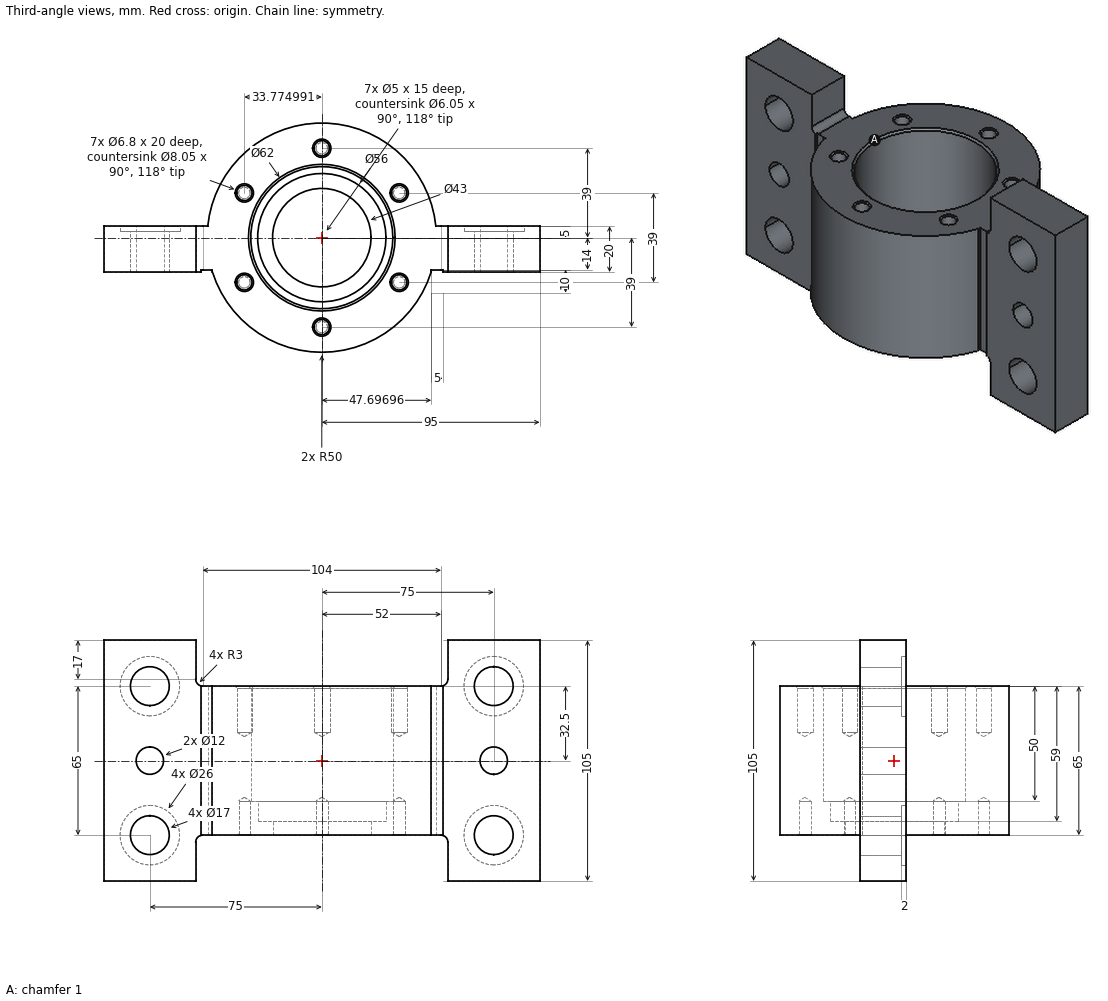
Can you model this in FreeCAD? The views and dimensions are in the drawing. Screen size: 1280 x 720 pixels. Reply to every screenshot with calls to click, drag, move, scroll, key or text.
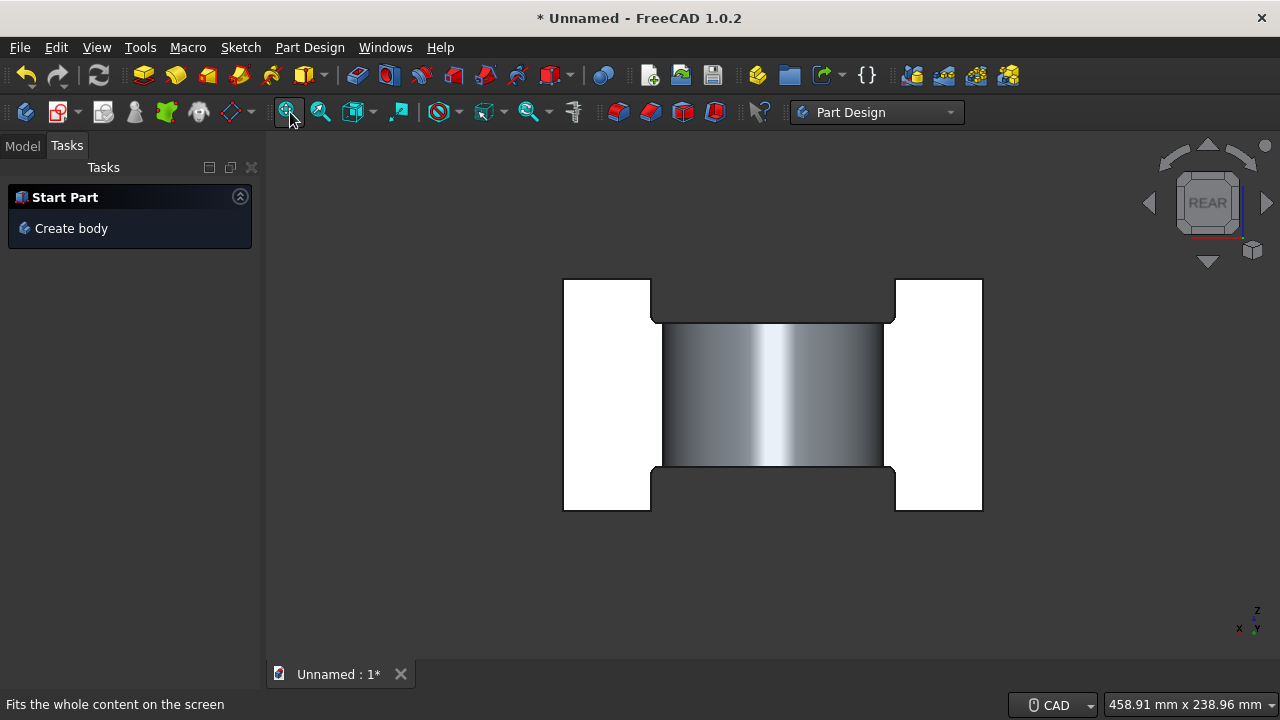
click(933, 361)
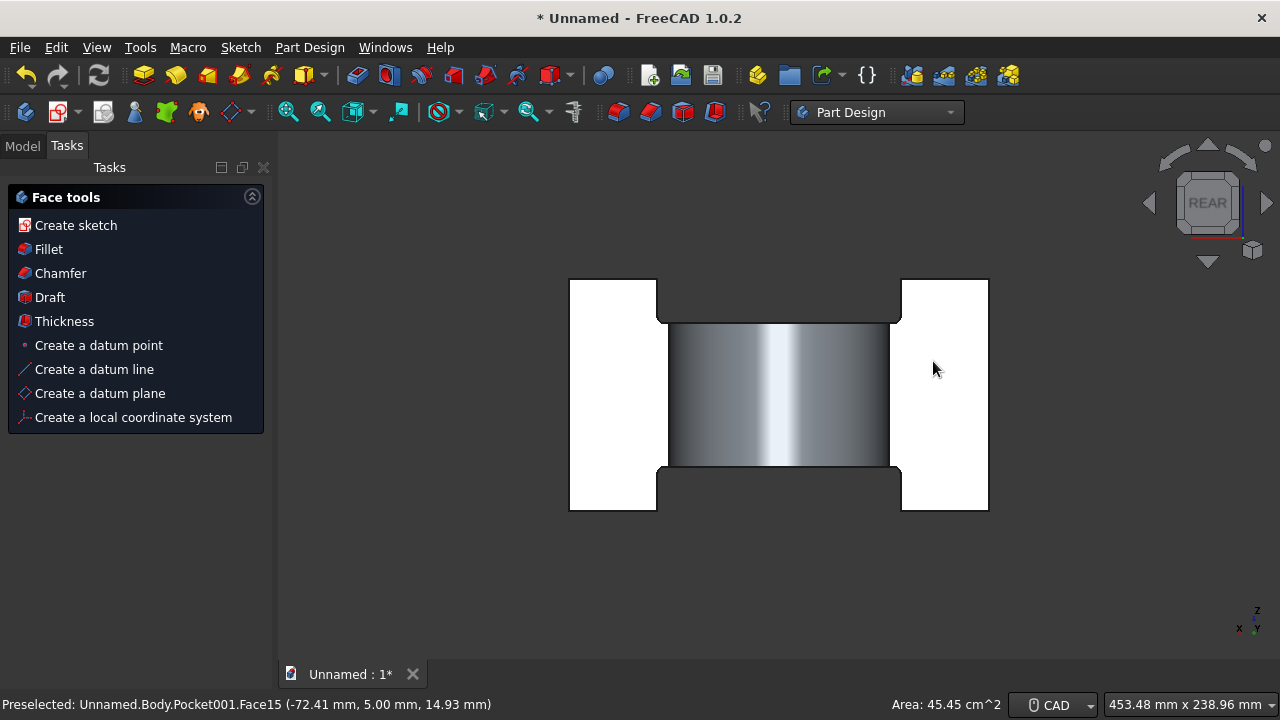
click(58, 112)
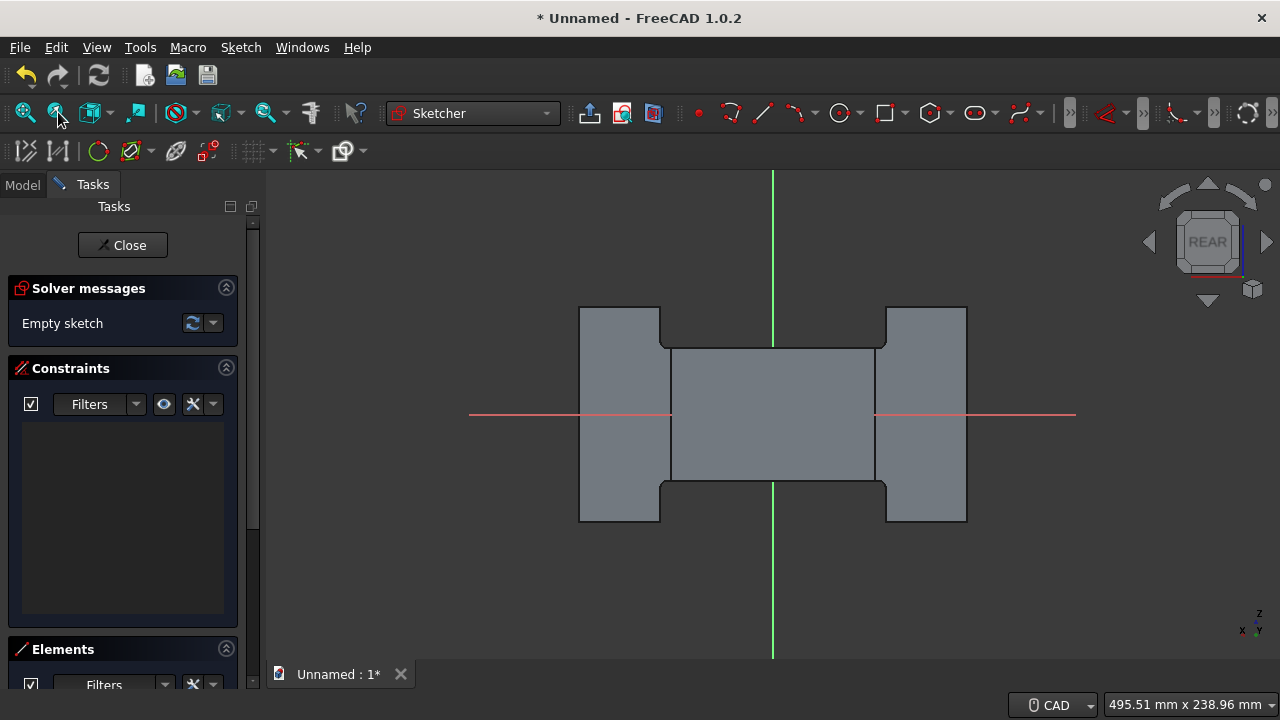
click(654, 114)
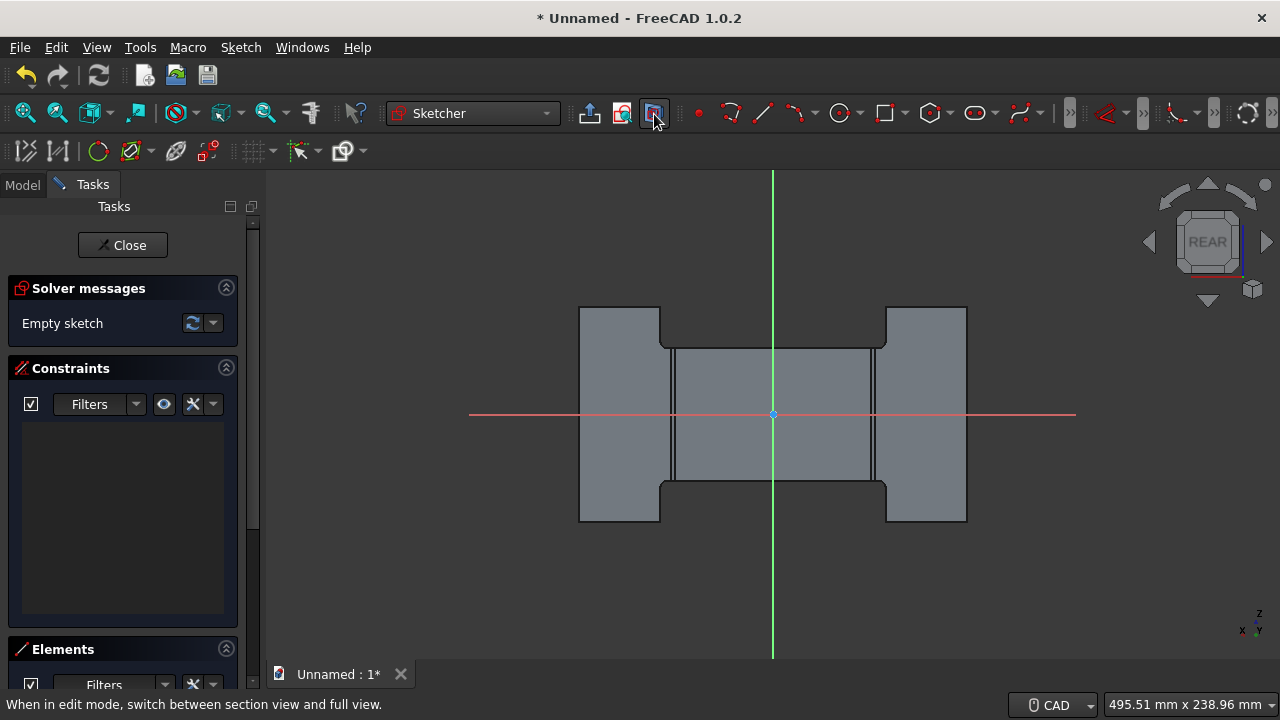
scroll(856, 415, up, 3)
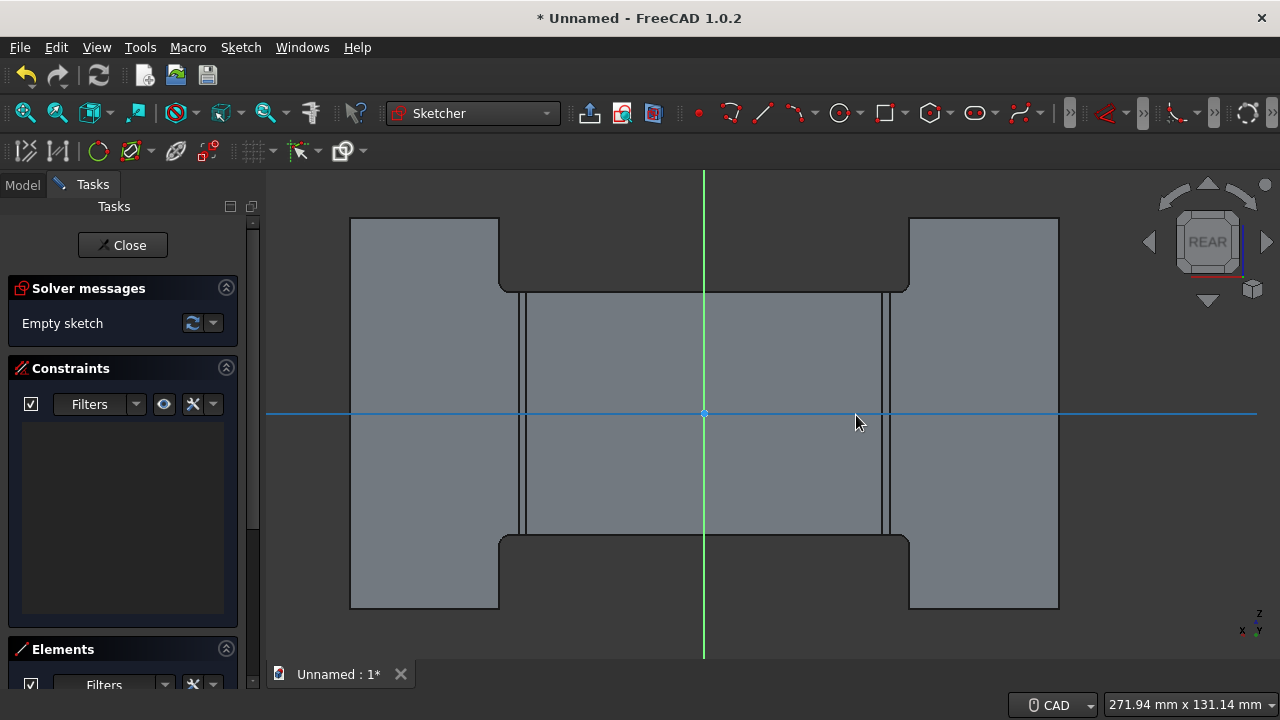
click(840, 114)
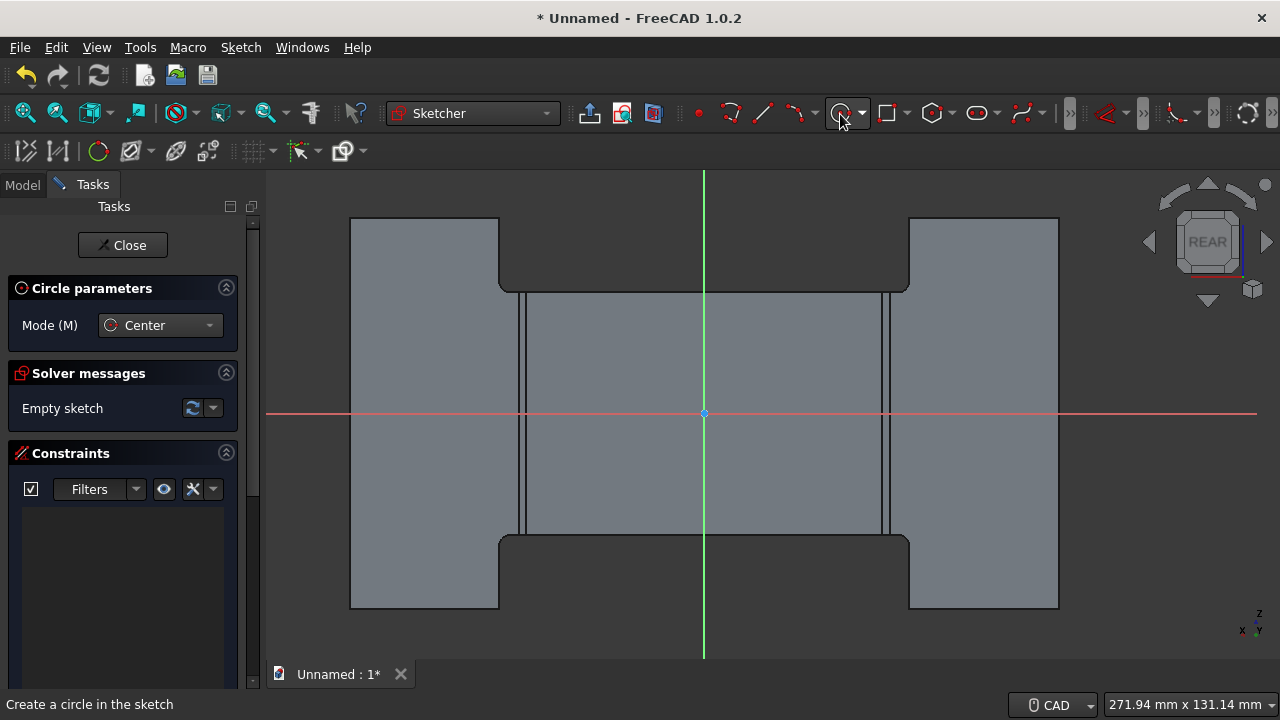
click(984, 535)
click(1006, 512)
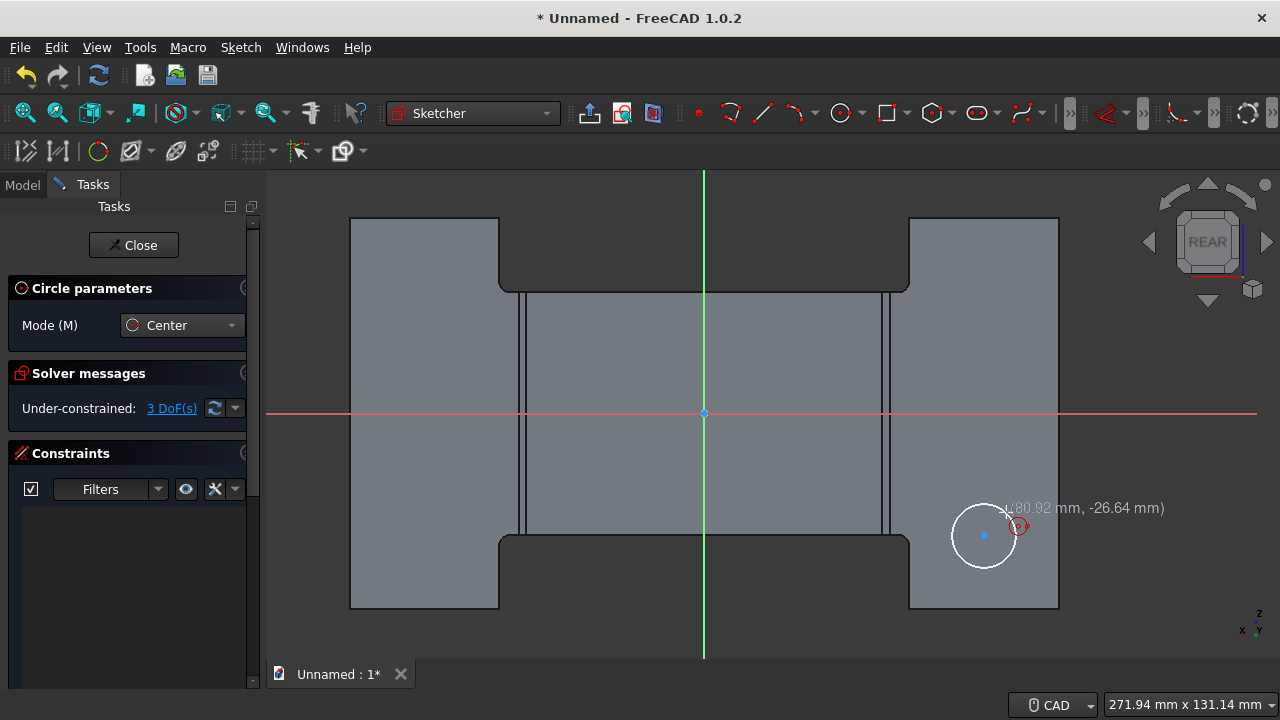
click(984, 292)
click(1006, 270)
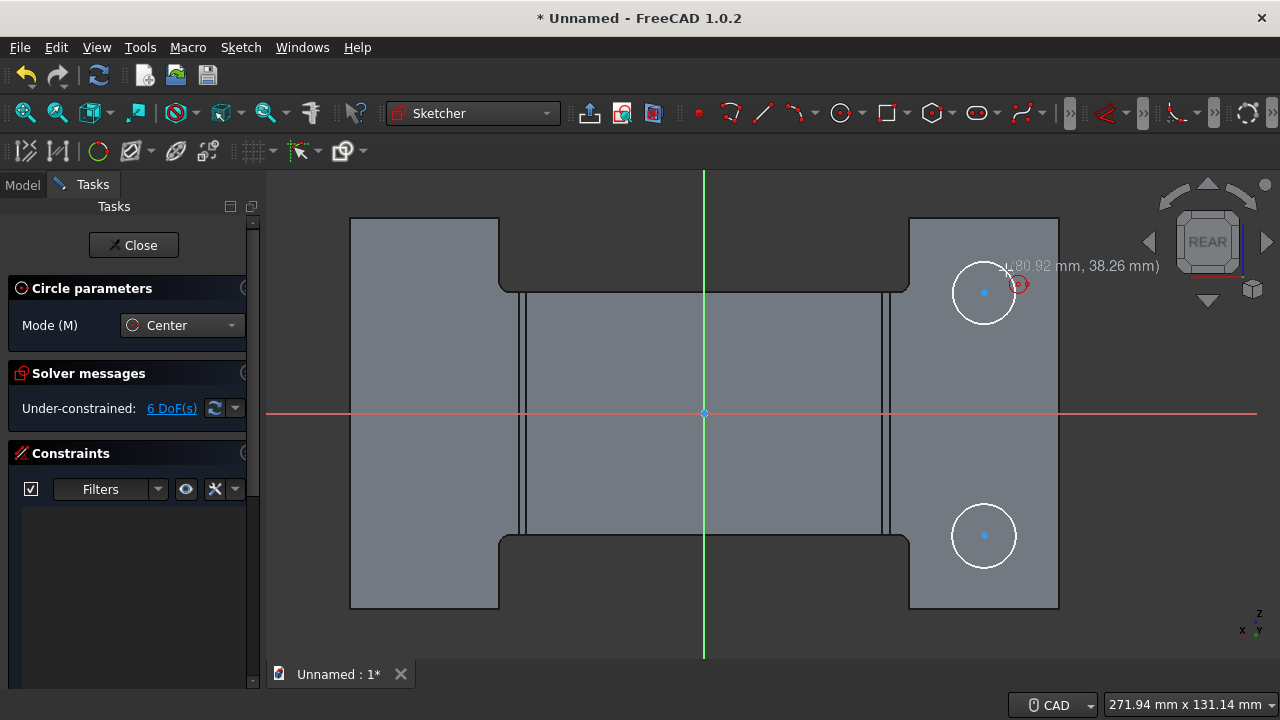
click(425, 292)
click(447, 270)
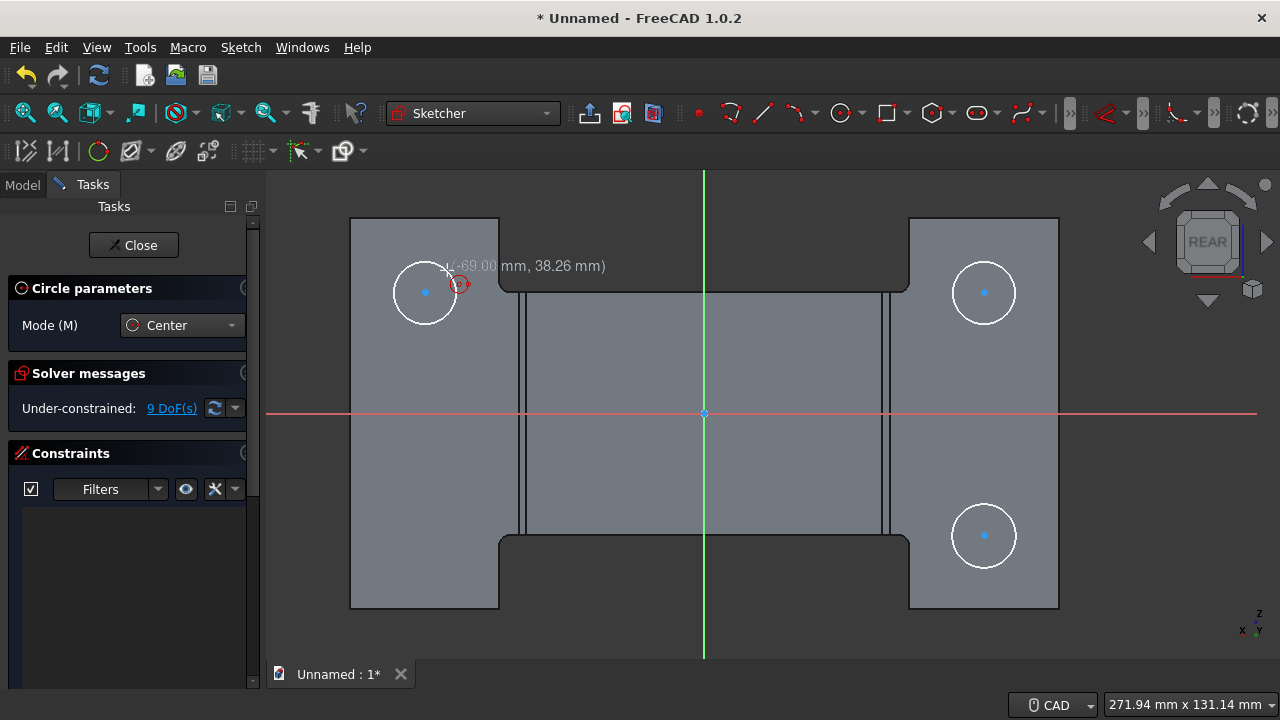
click(425, 535)
click(447, 512)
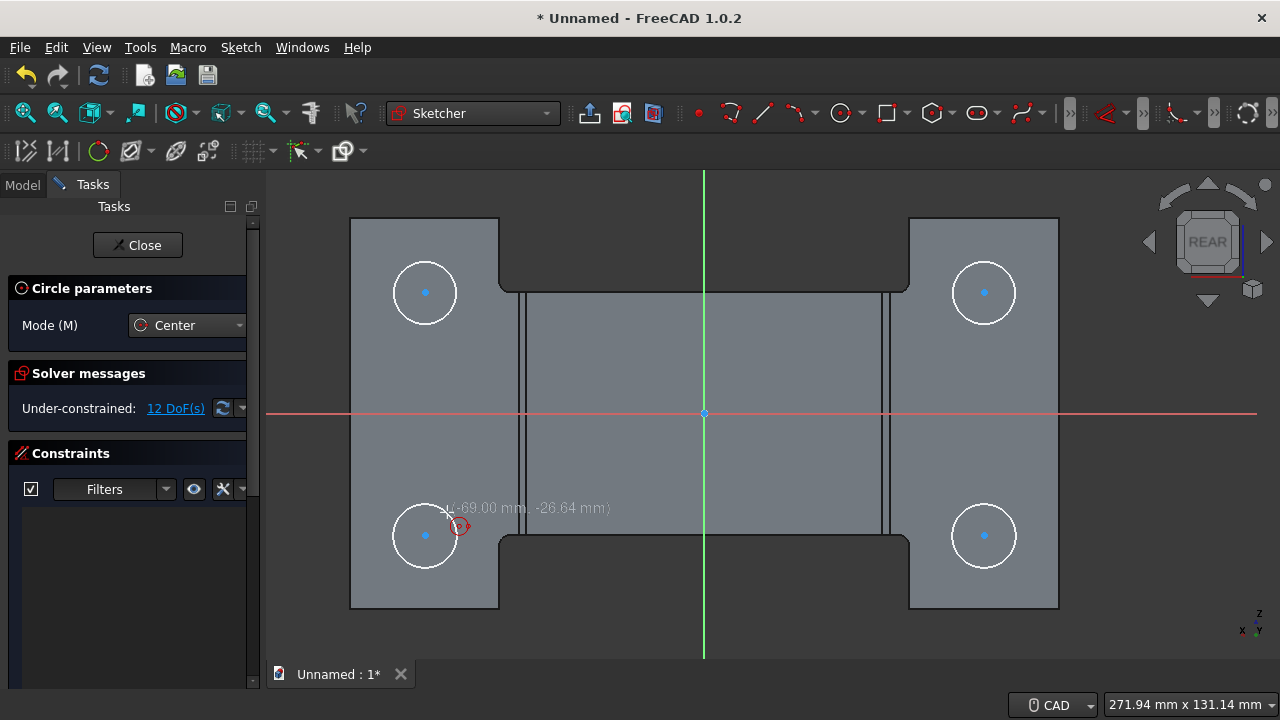
click(984, 414)
click(1000, 398)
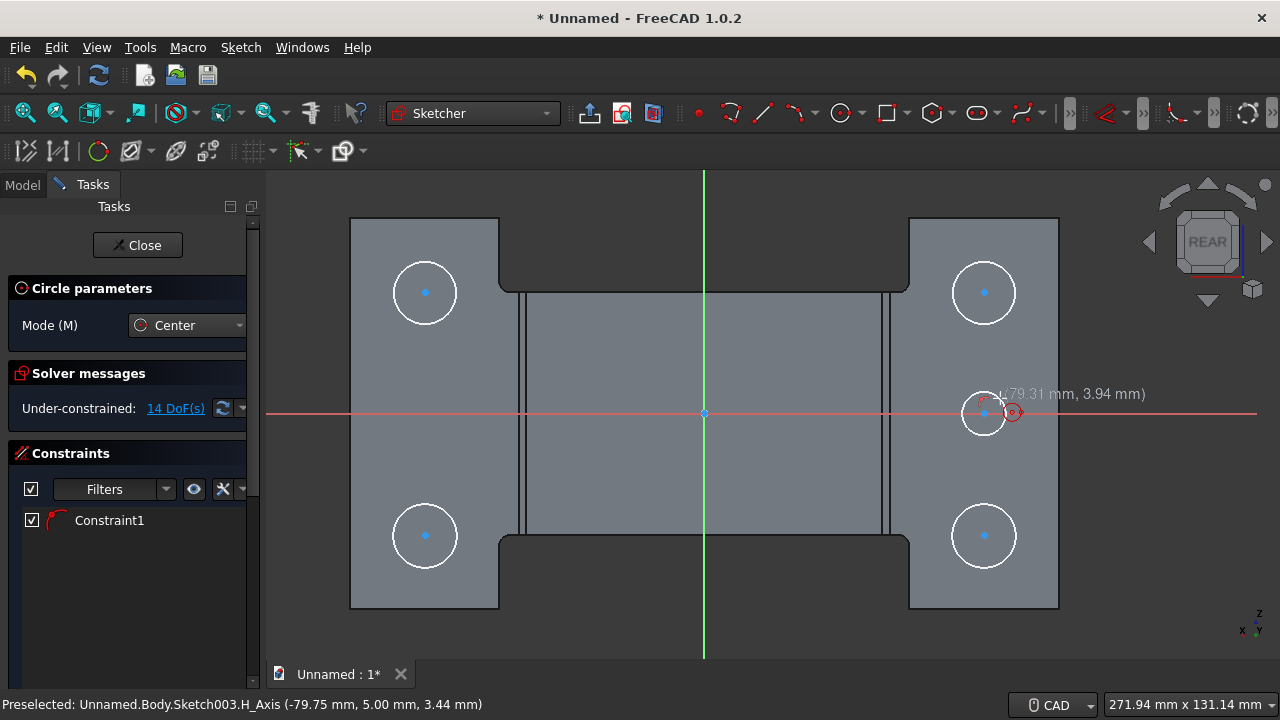
click(425, 414)
click(440, 398)
key(Escape)